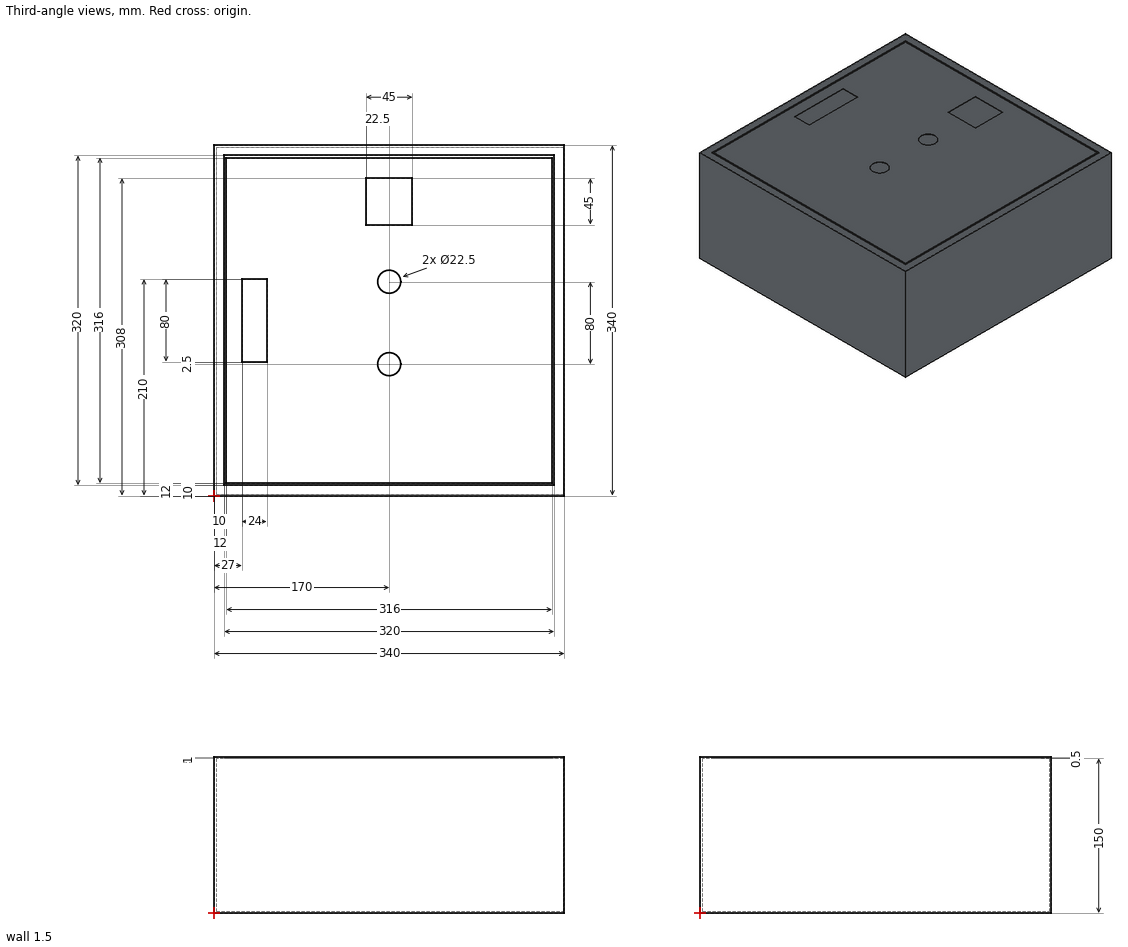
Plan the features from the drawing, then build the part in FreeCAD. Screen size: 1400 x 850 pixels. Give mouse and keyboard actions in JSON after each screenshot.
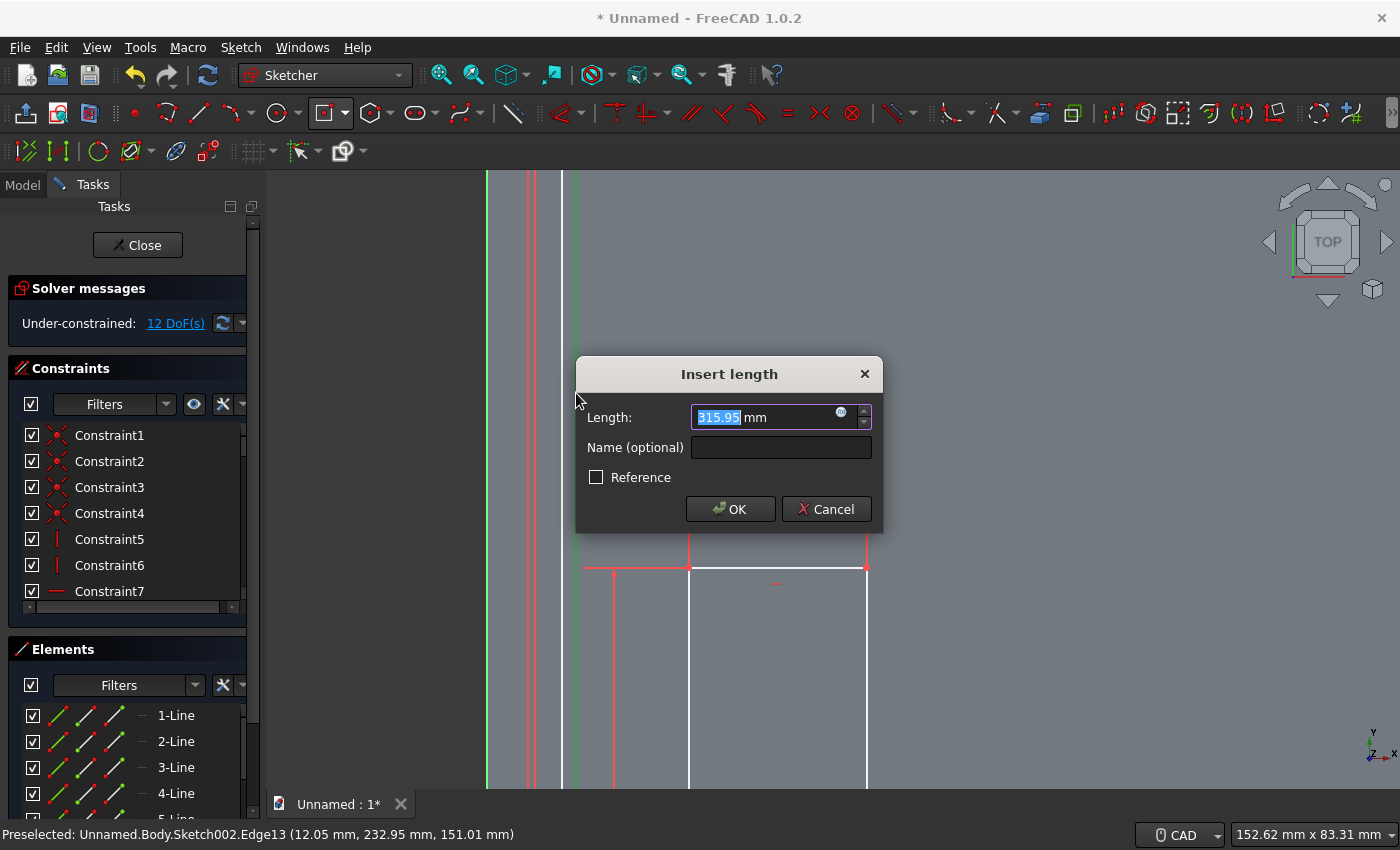
{"action": "type", "text": "316"}
{"action": "key", "text": "Return"}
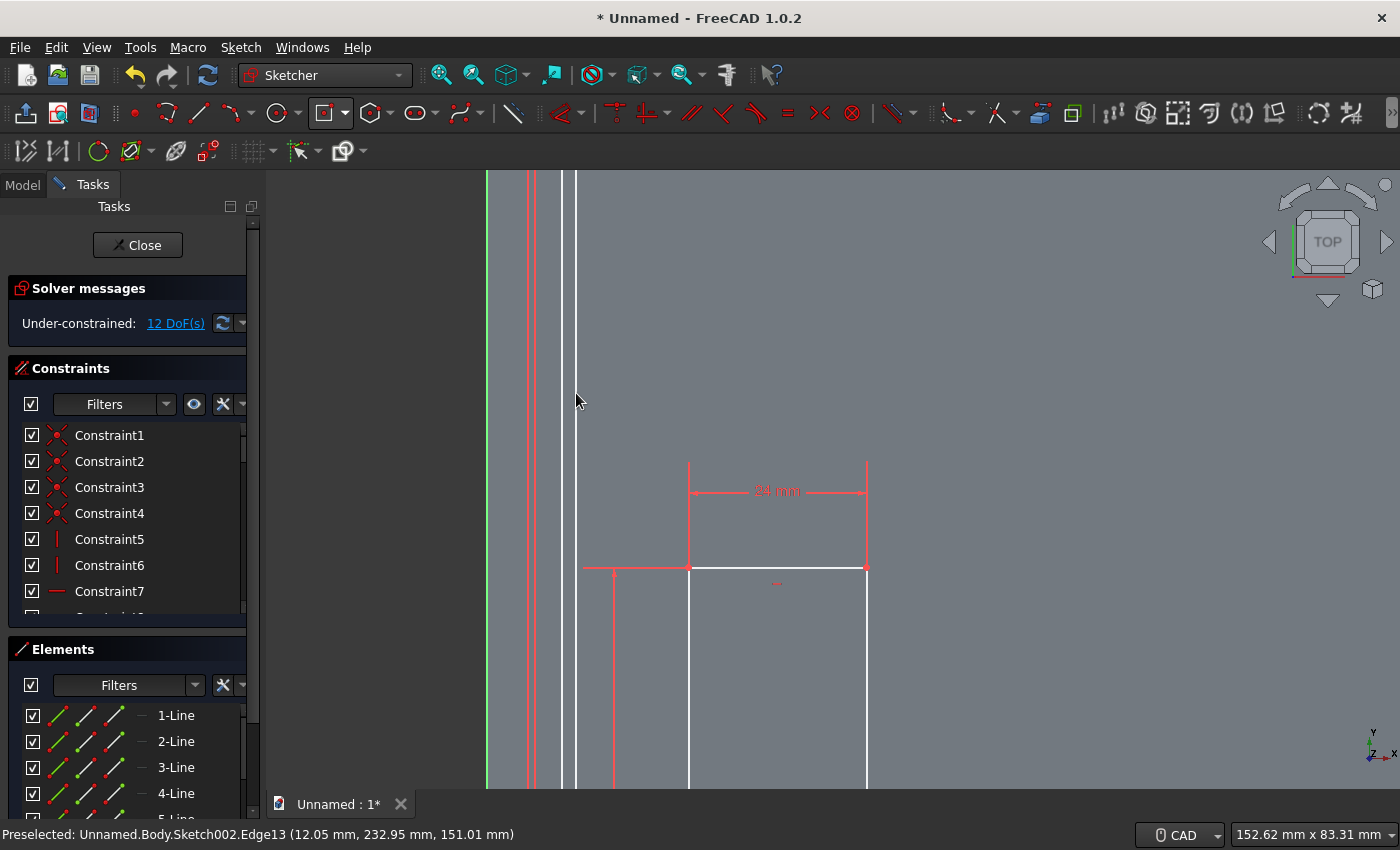
{"action": "scroll", "coordinate": [577, 396], "scroll_direction": "down", "scroll_amount": 9}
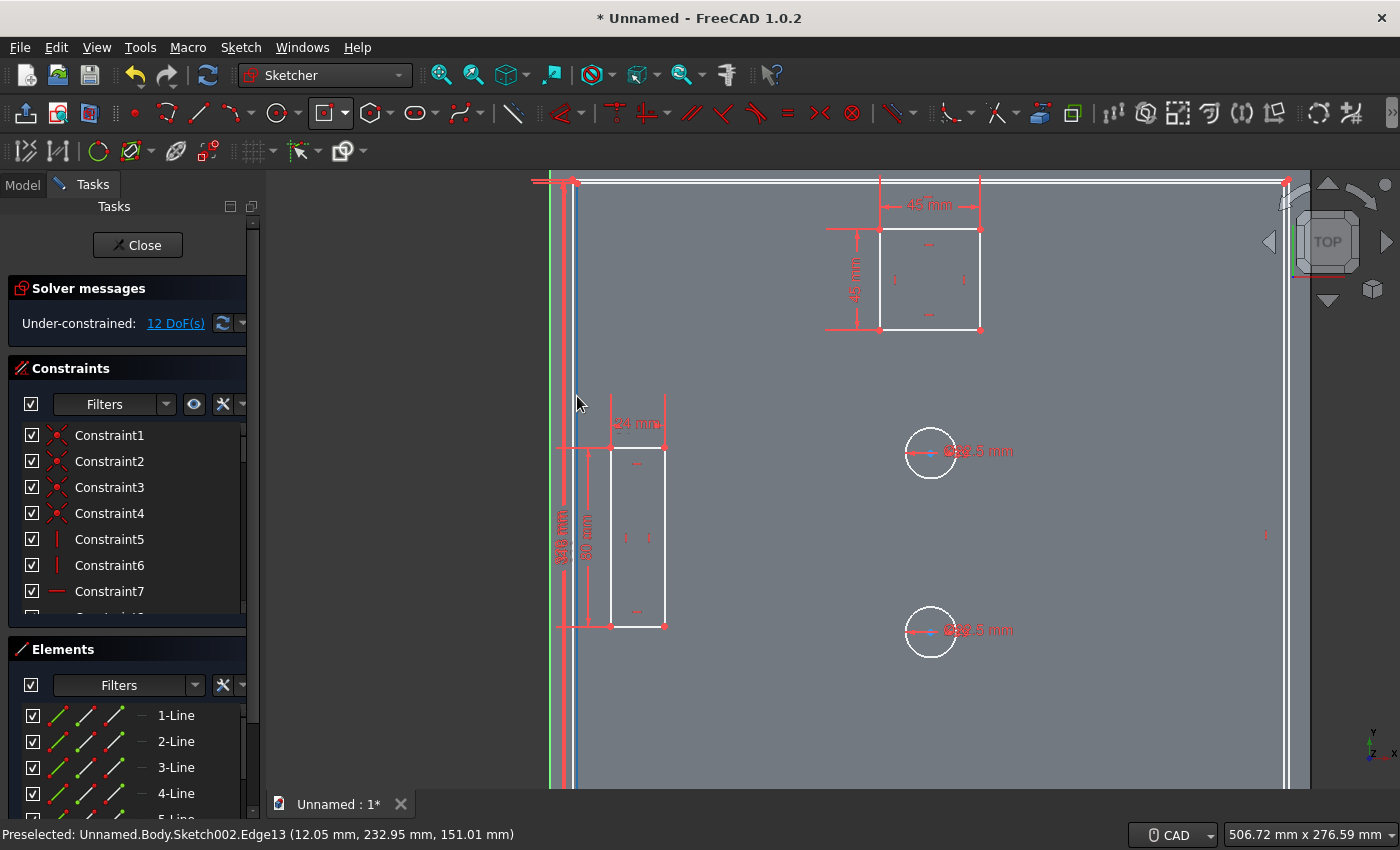
{"action": "scroll", "coordinate": [694, 668], "scroll_direction": "up", "scroll_amount": 8}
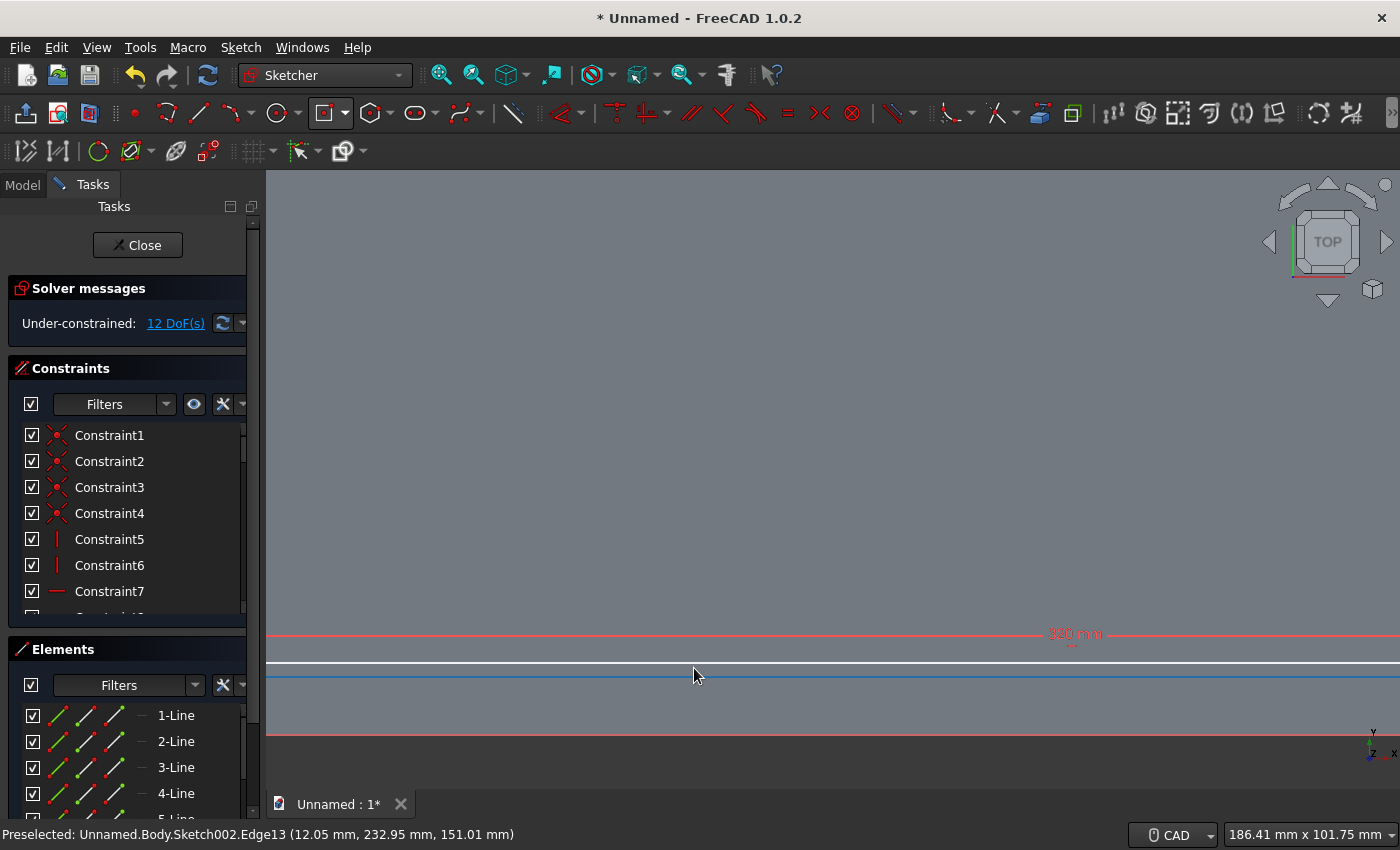
{"action": "left_click", "coordinate": [690, 663]}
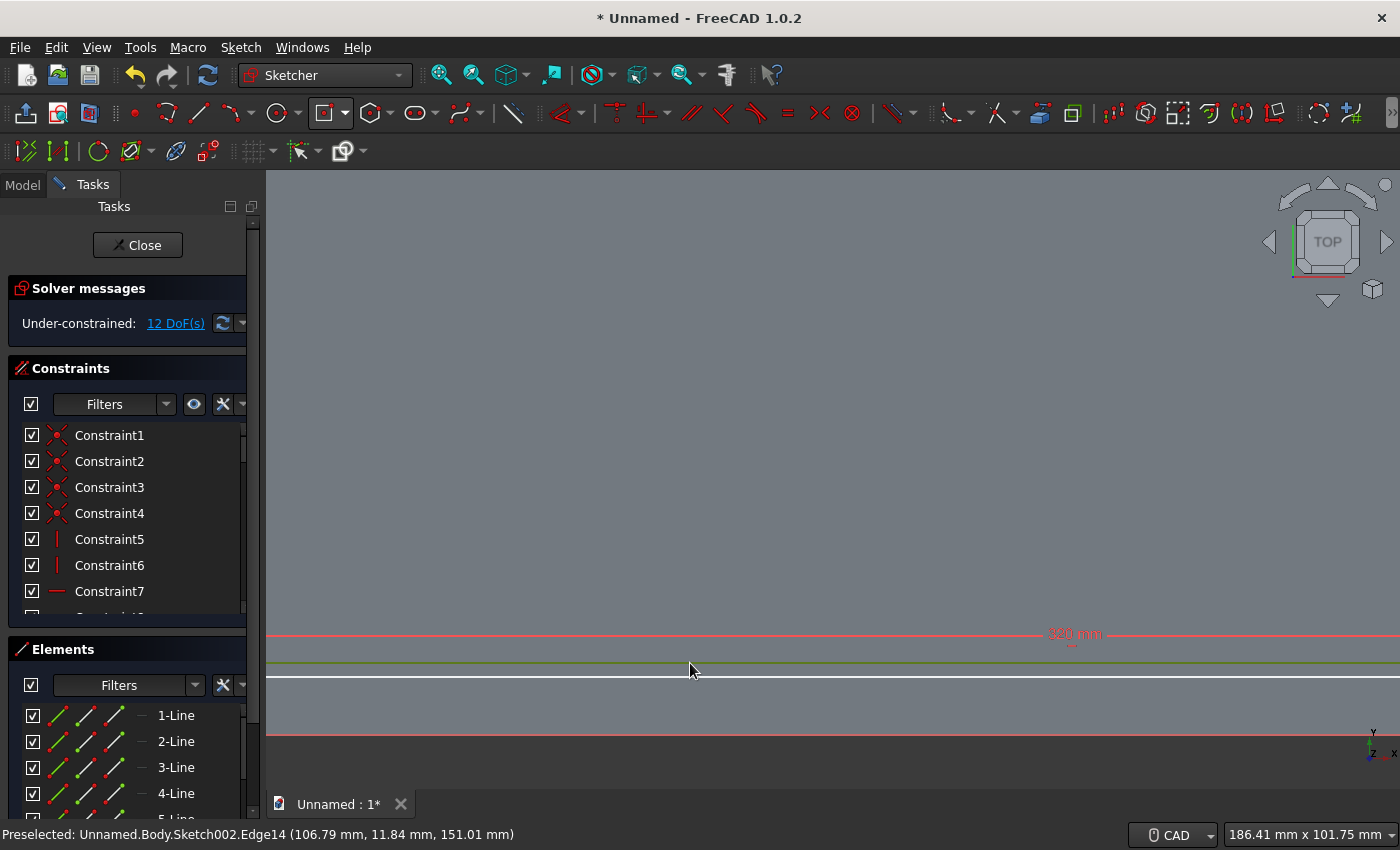
{"action": "key", "text": "l"}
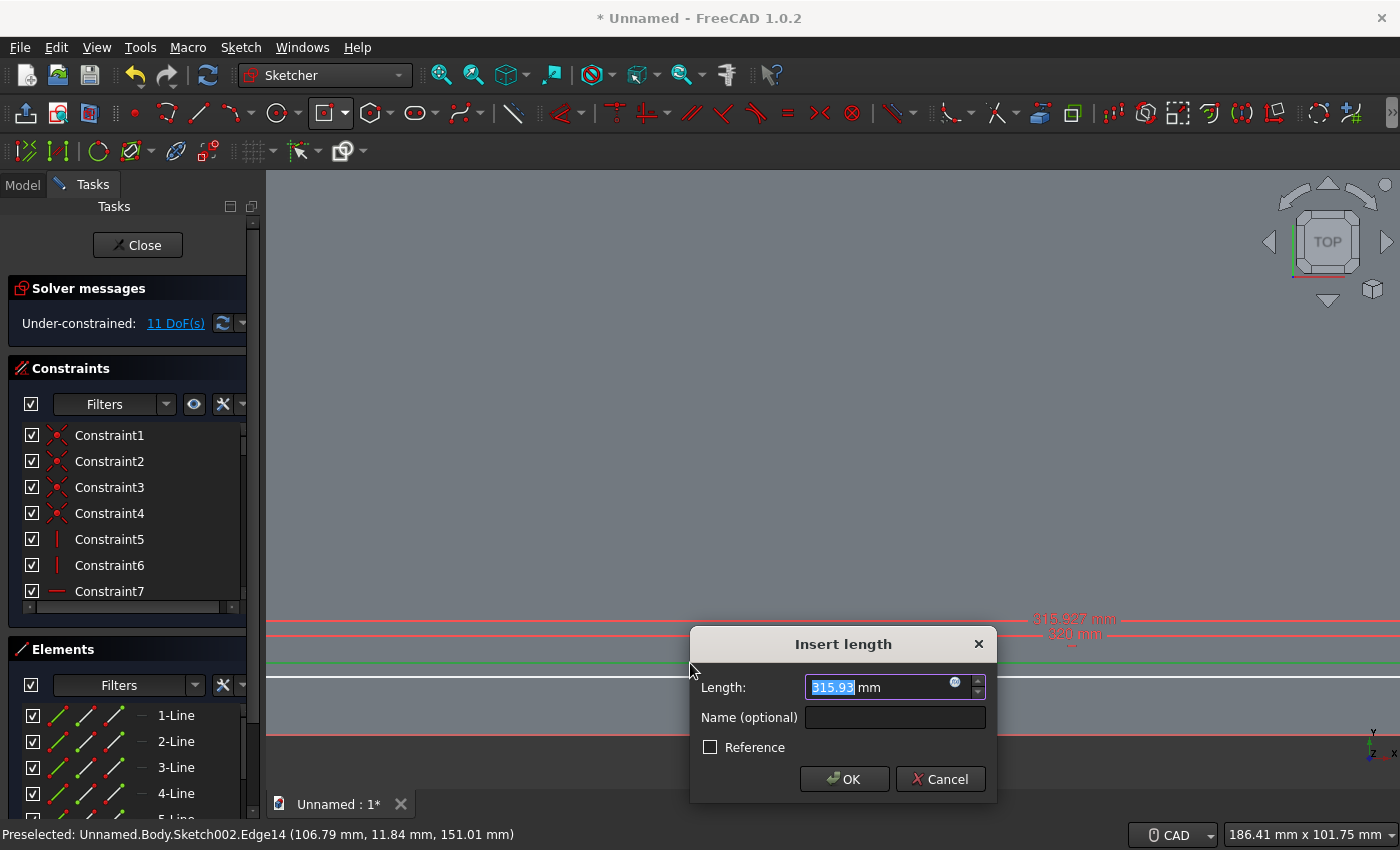
{"action": "type", "text": "316"}
{"action": "key", "text": "Return"}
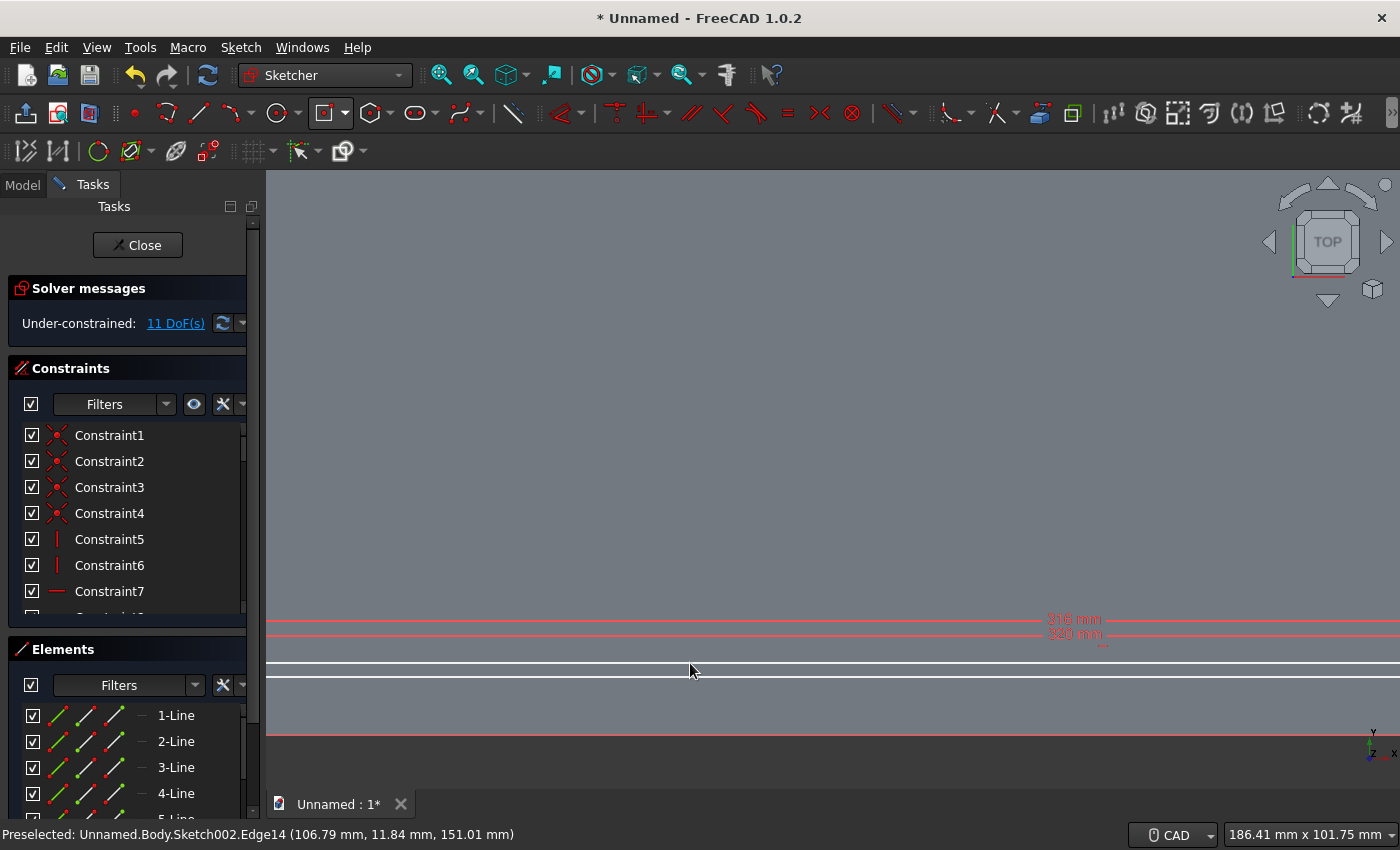
{"action": "scroll", "coordinate": [694, 669], "scroll_direction": "down", "scroll_amount": 8}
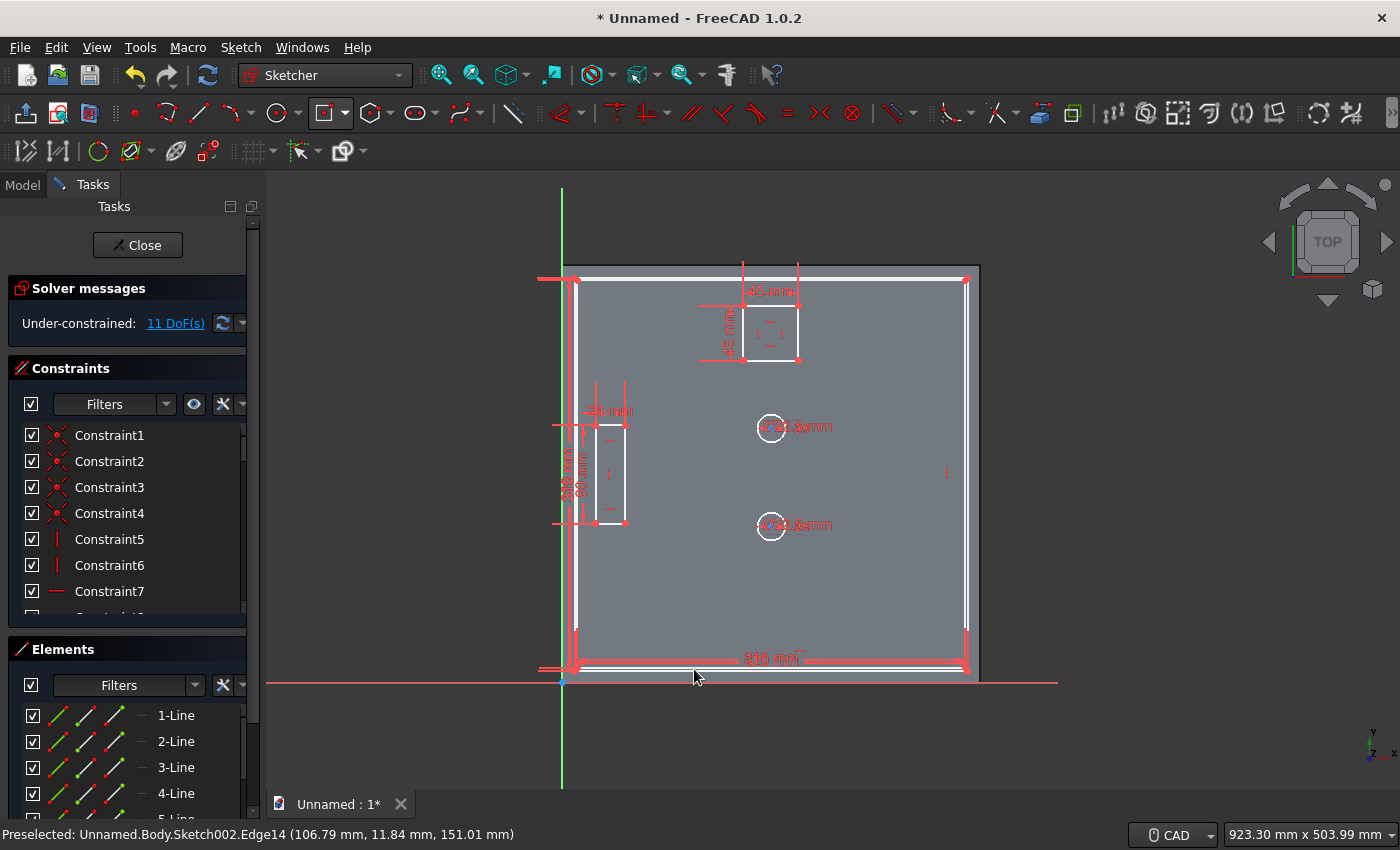
{"action": "scroll", "coordinate": [575, 278], "scroll_direction": "up", "scroll_amount": 8}